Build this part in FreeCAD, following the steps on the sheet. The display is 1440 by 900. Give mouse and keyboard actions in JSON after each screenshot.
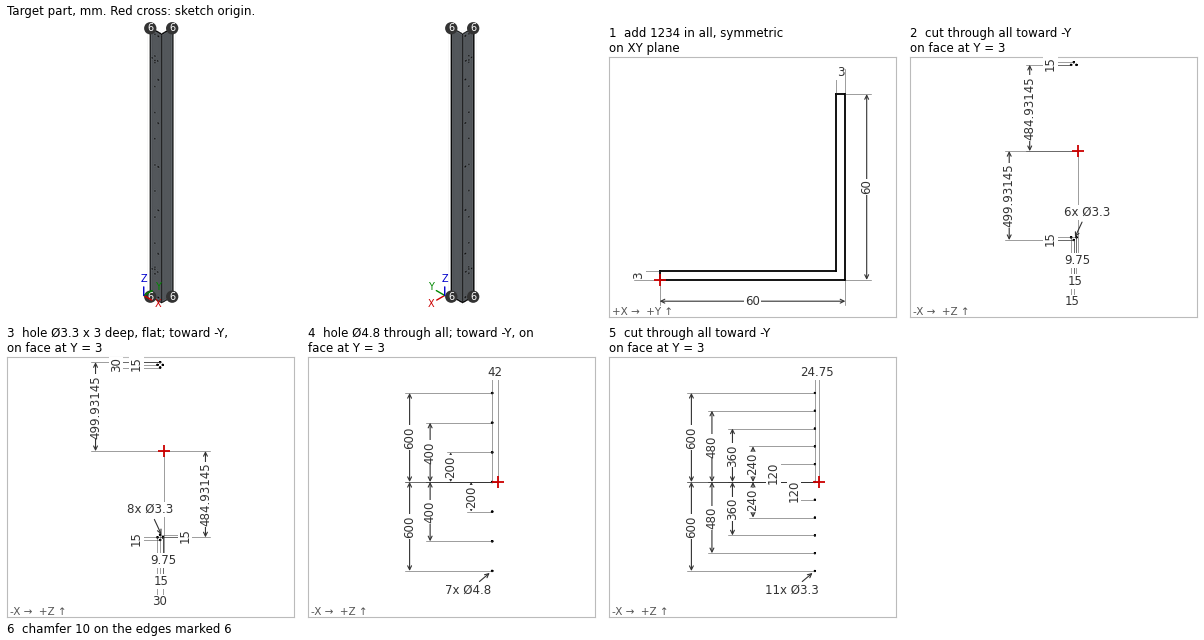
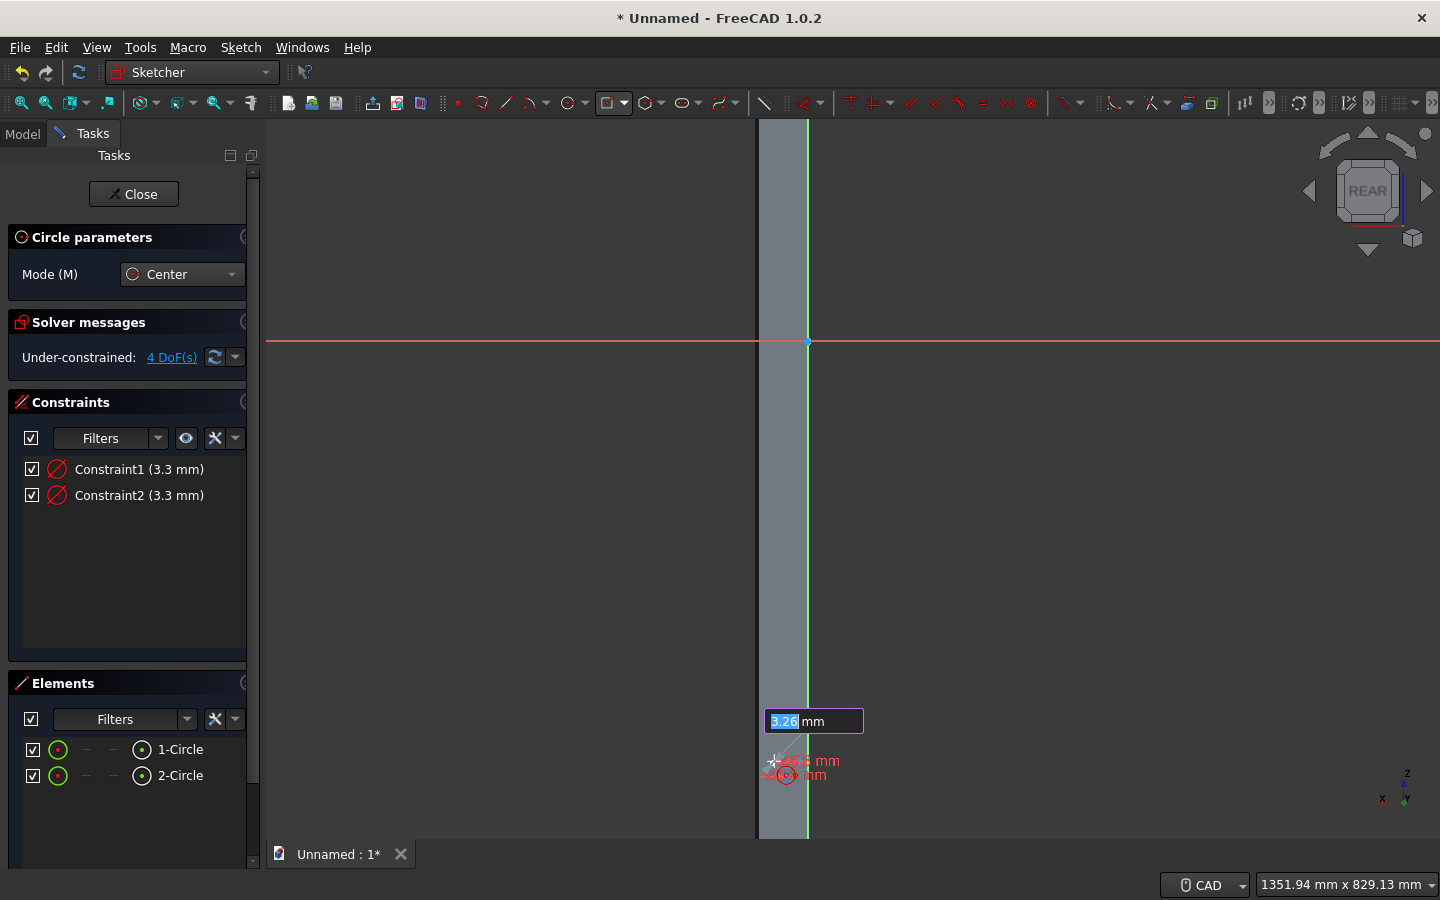
{"action": "type", "text": "3.3"}
{"action": "key", "text": "Return"}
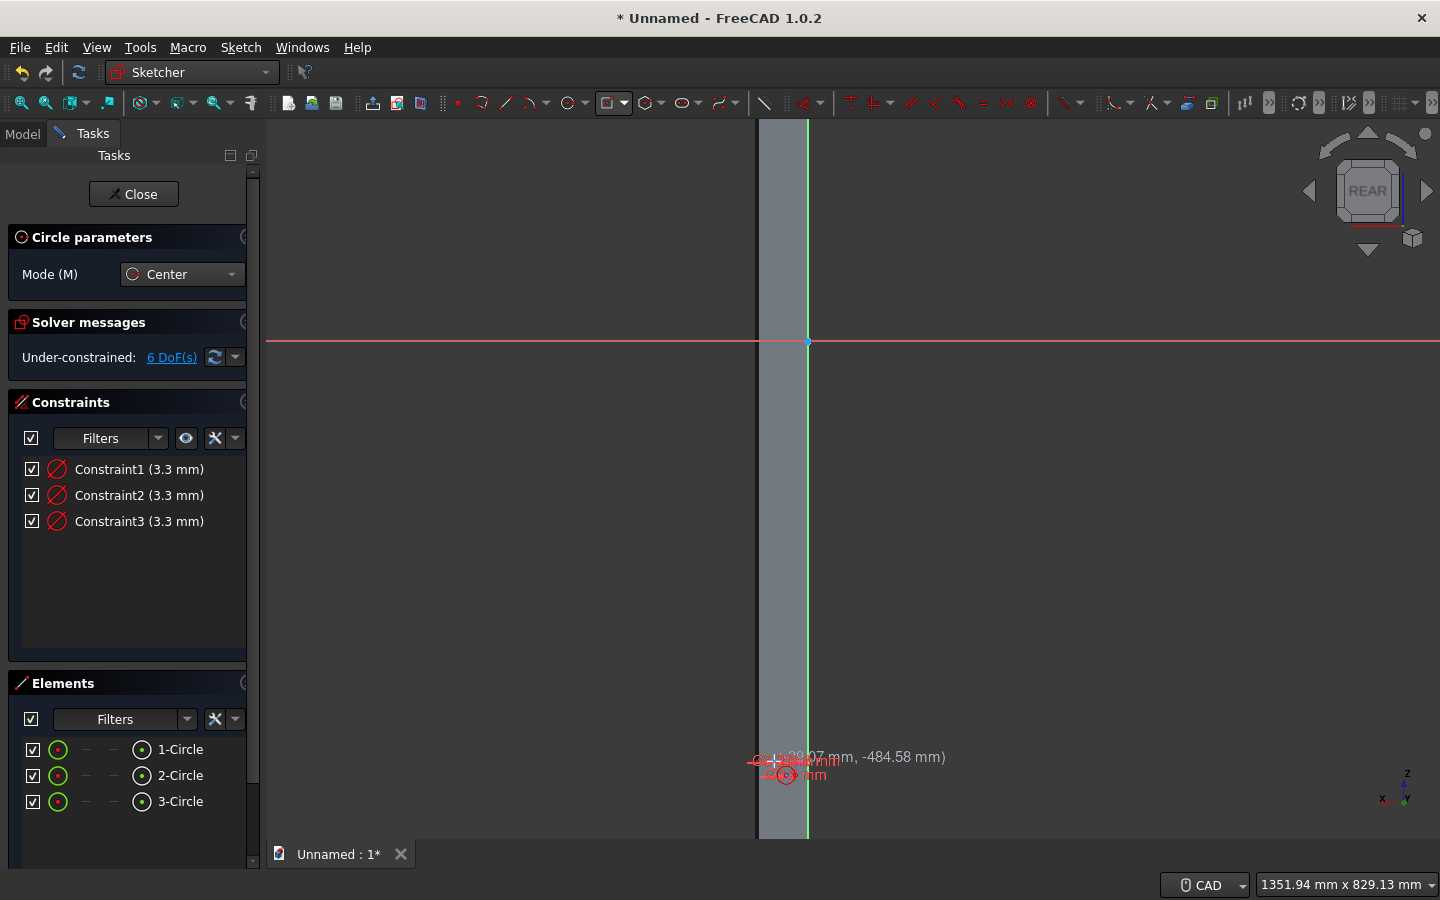
{"action": "scroll", "coordinate": [778, 647], "scroll_direction": "down", "scroll_amount": 3}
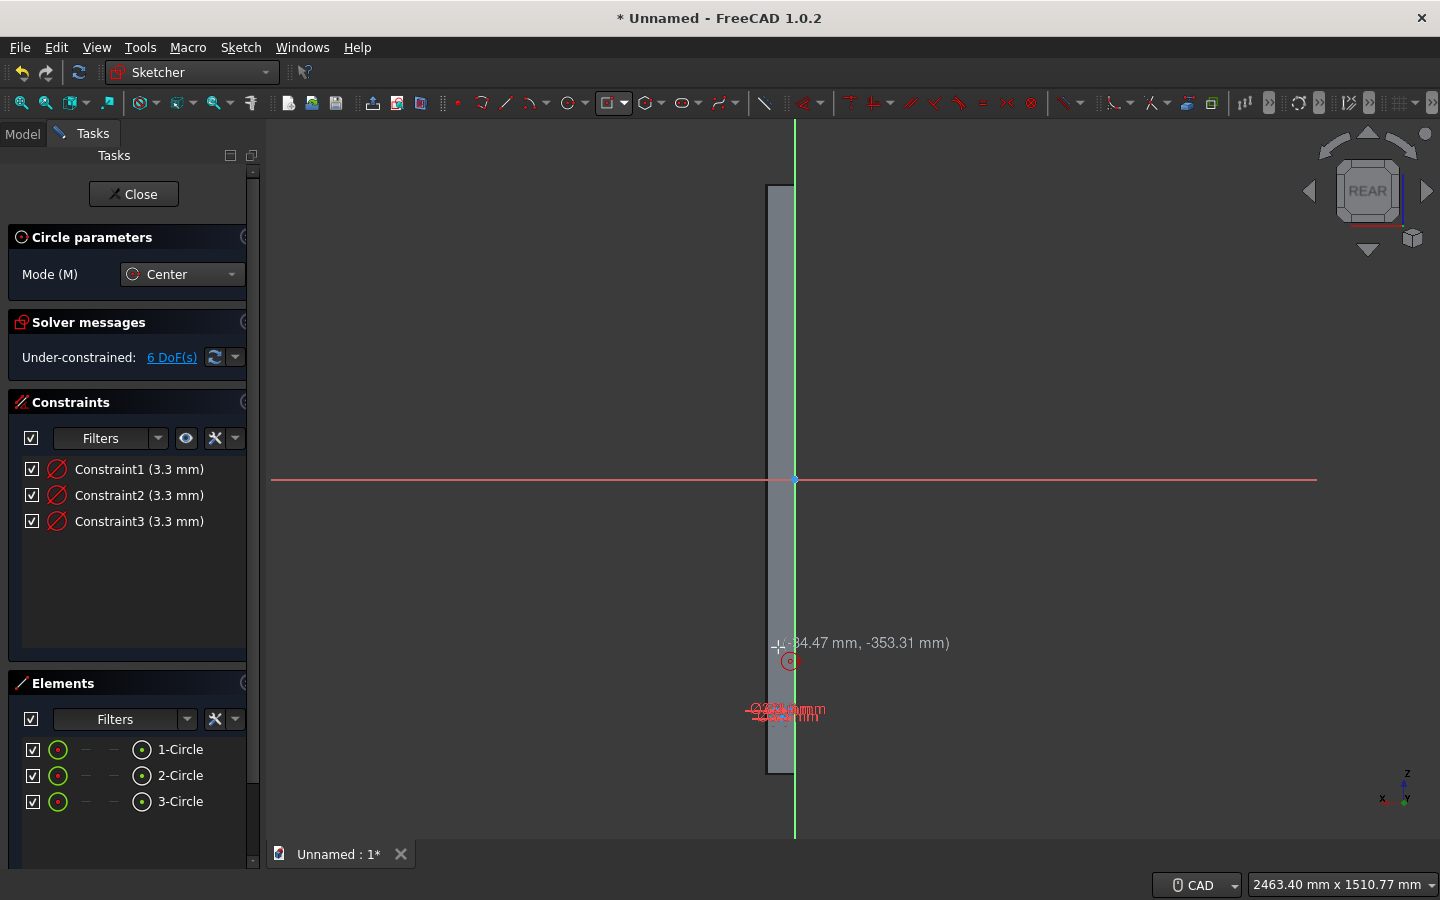
{"action": "scroll", "coordinate": [776, 248], "scroll_direction": "up", "scroll_amount": 17}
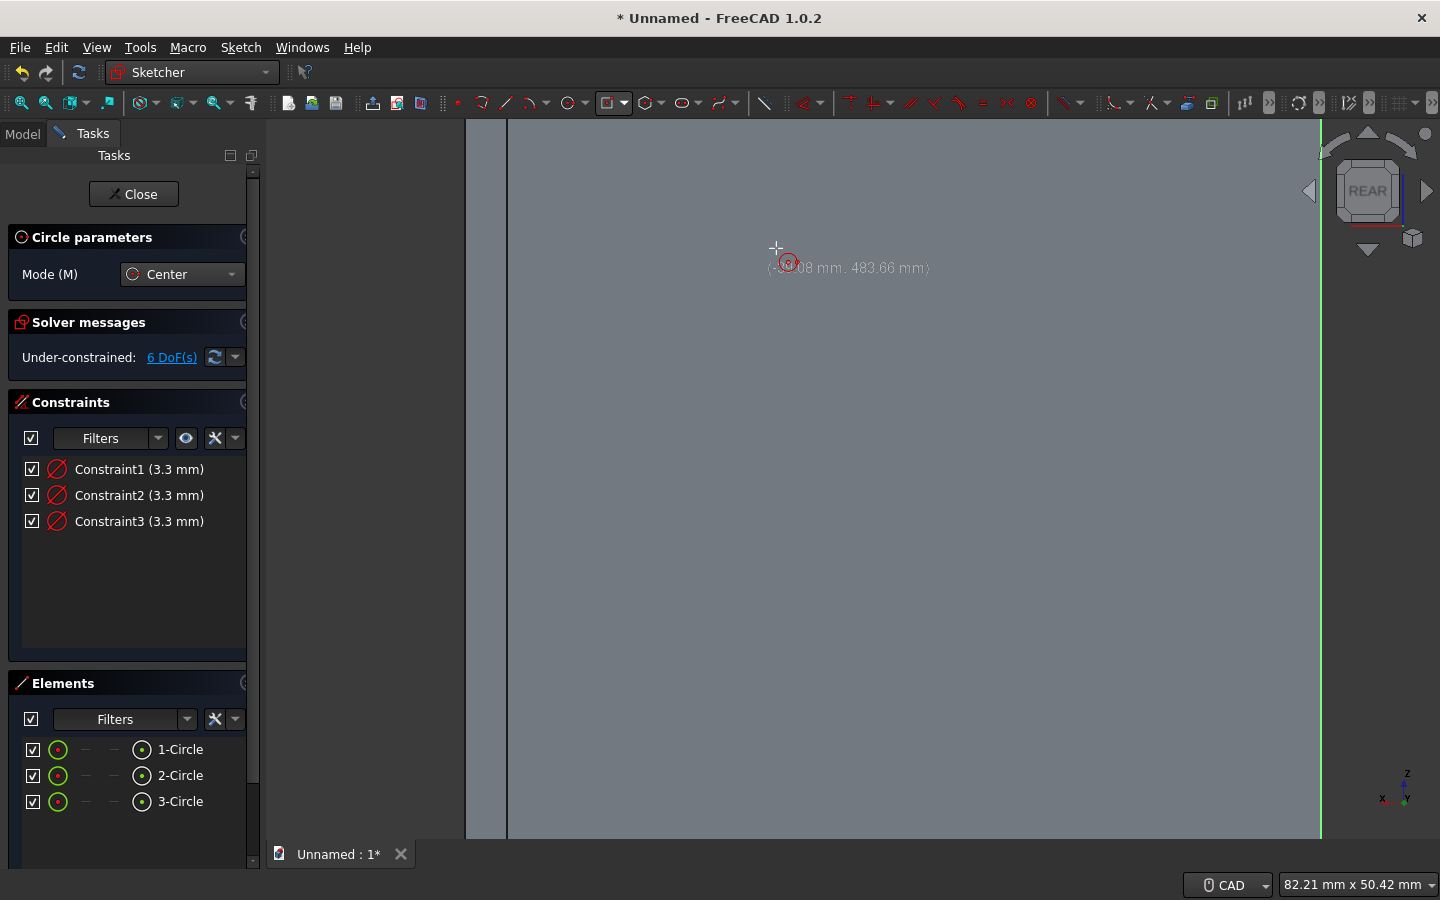
{"action": "scroll", "coordinate": [774, 194], "scroll_direction": "down", "scroll_amount": 16}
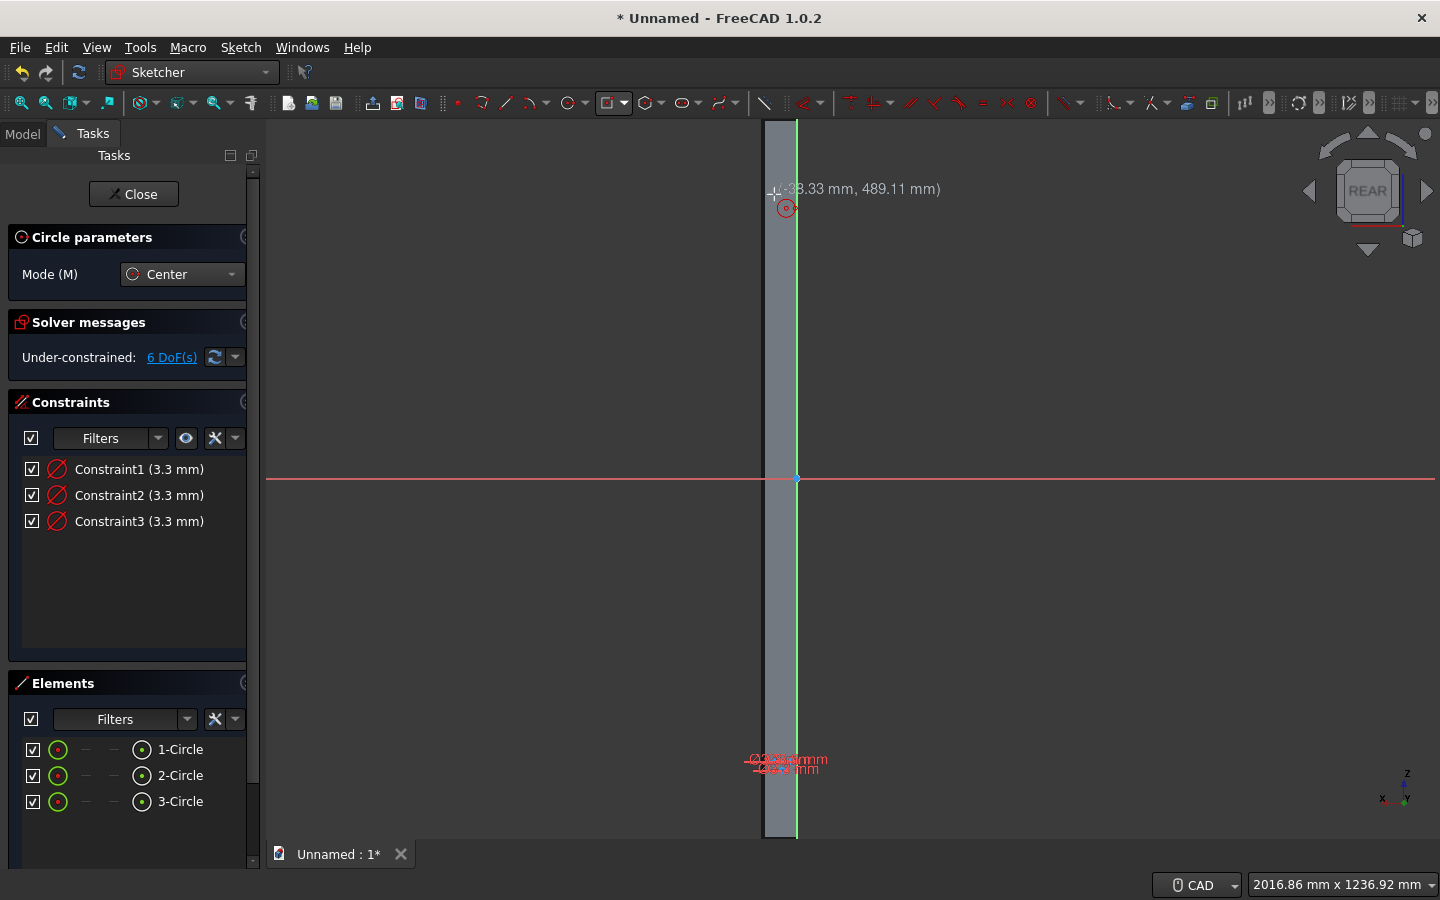
{"action": "left_click", "coordinate": [774, 197]}
{"action": "mouse_move", "coordinate": [774, 196]}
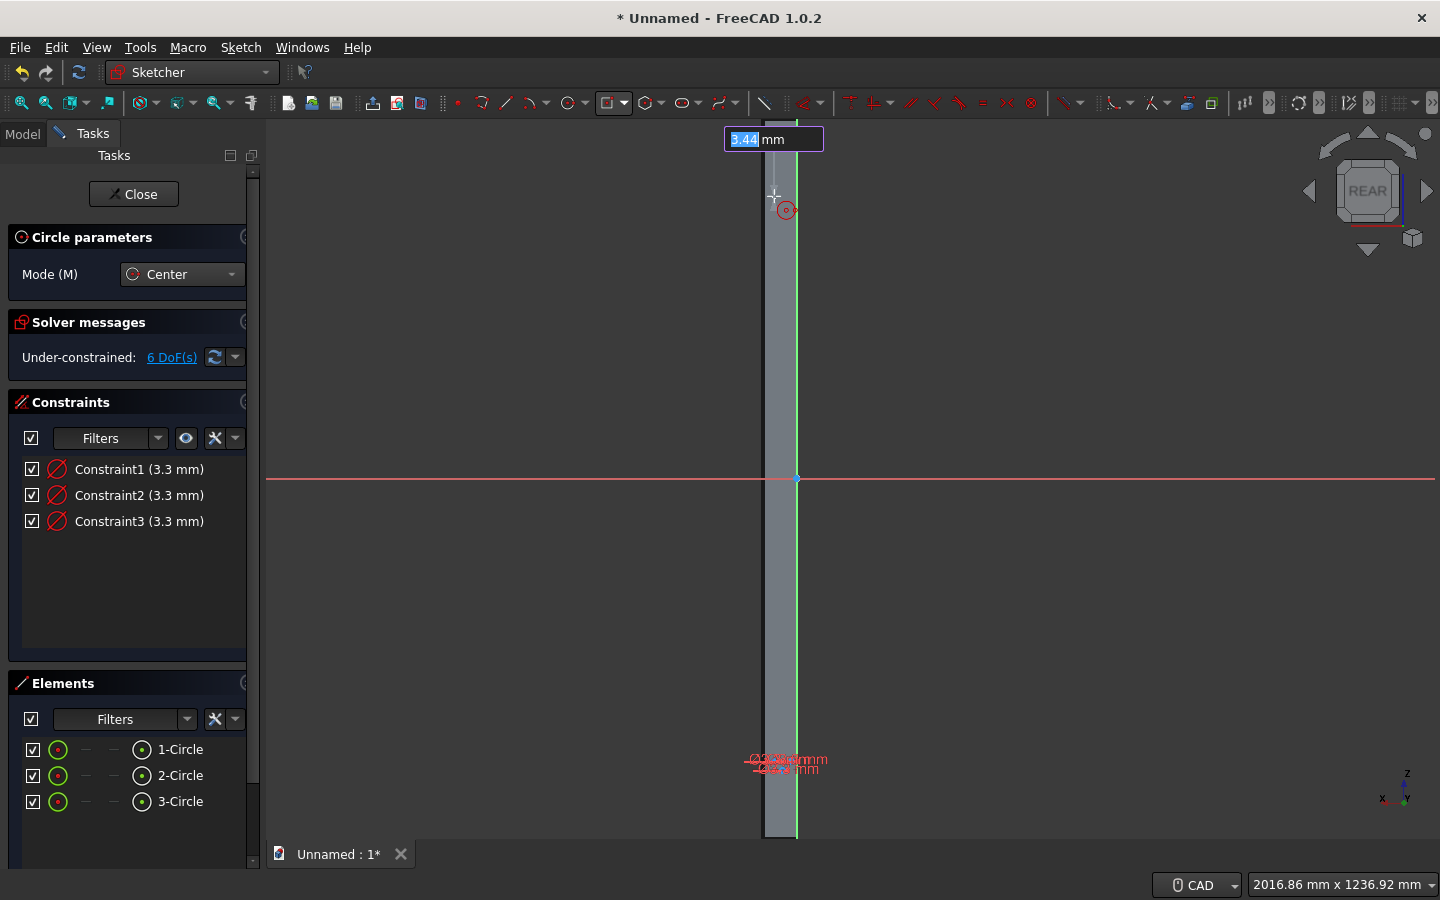
{"action": "type", "text": "3.3"}
{"action": "key", "text": "Return"}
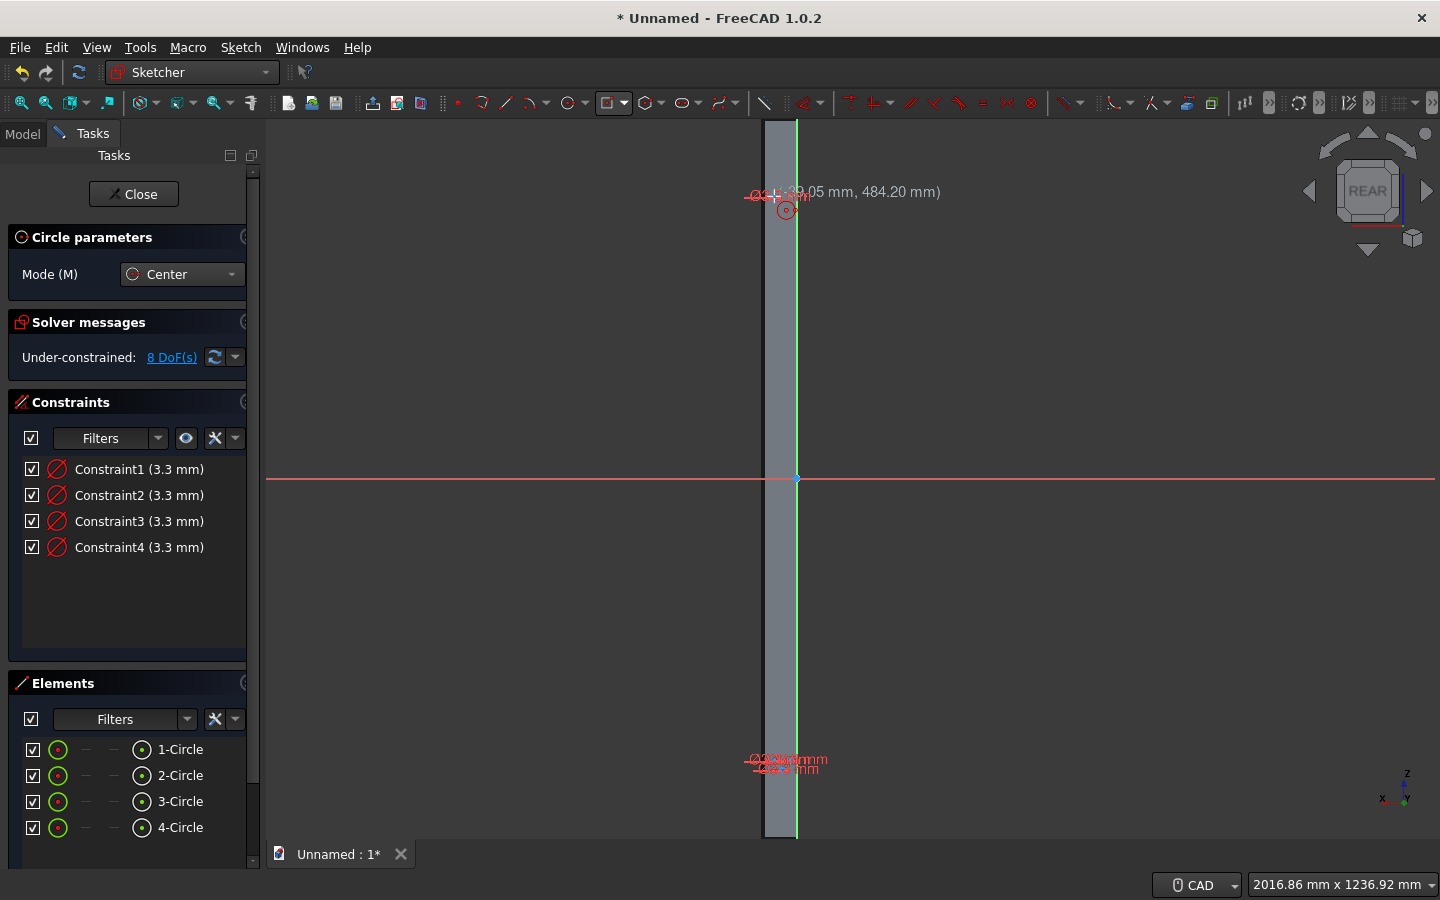
{"action": "scroll", "coordinate": [791, 197], "scroll_direction": "up", "scroll_amount": 16}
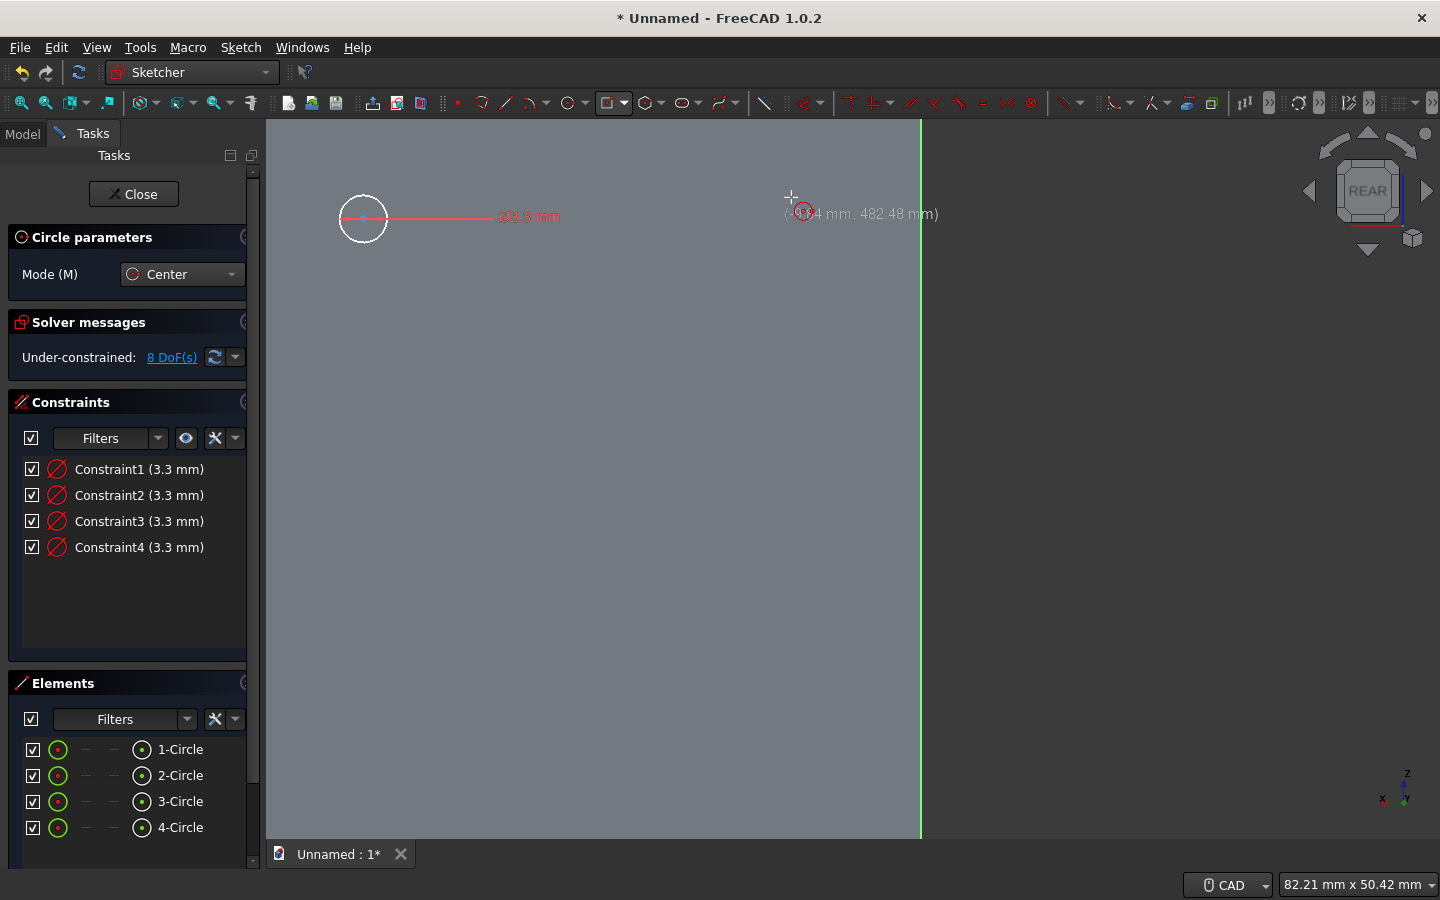
{"action": "scroll", "coordinate": [791, 197], "scroll_direction": "down", "scroll_amount": 16}